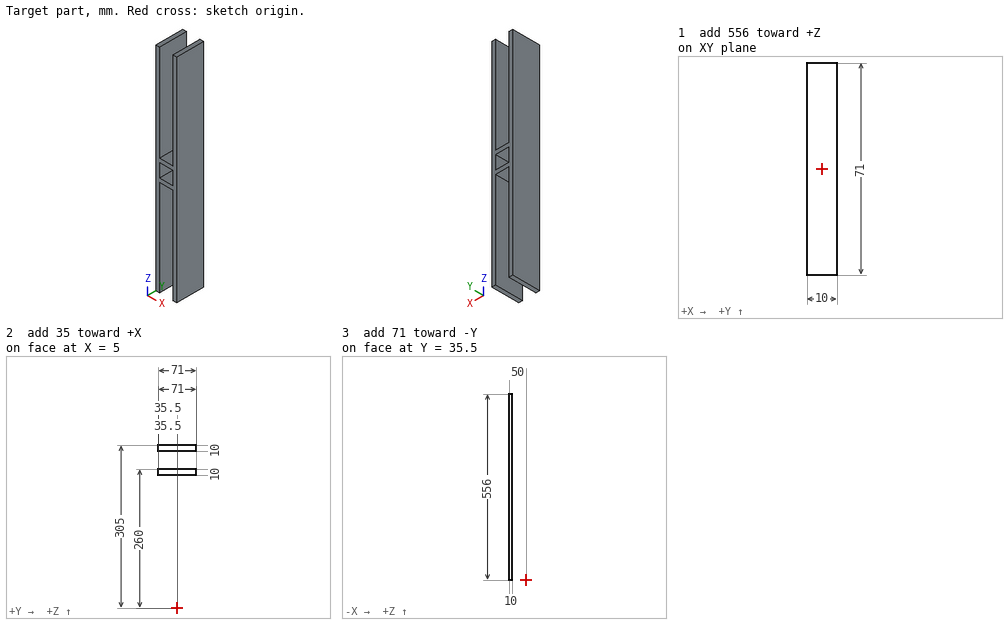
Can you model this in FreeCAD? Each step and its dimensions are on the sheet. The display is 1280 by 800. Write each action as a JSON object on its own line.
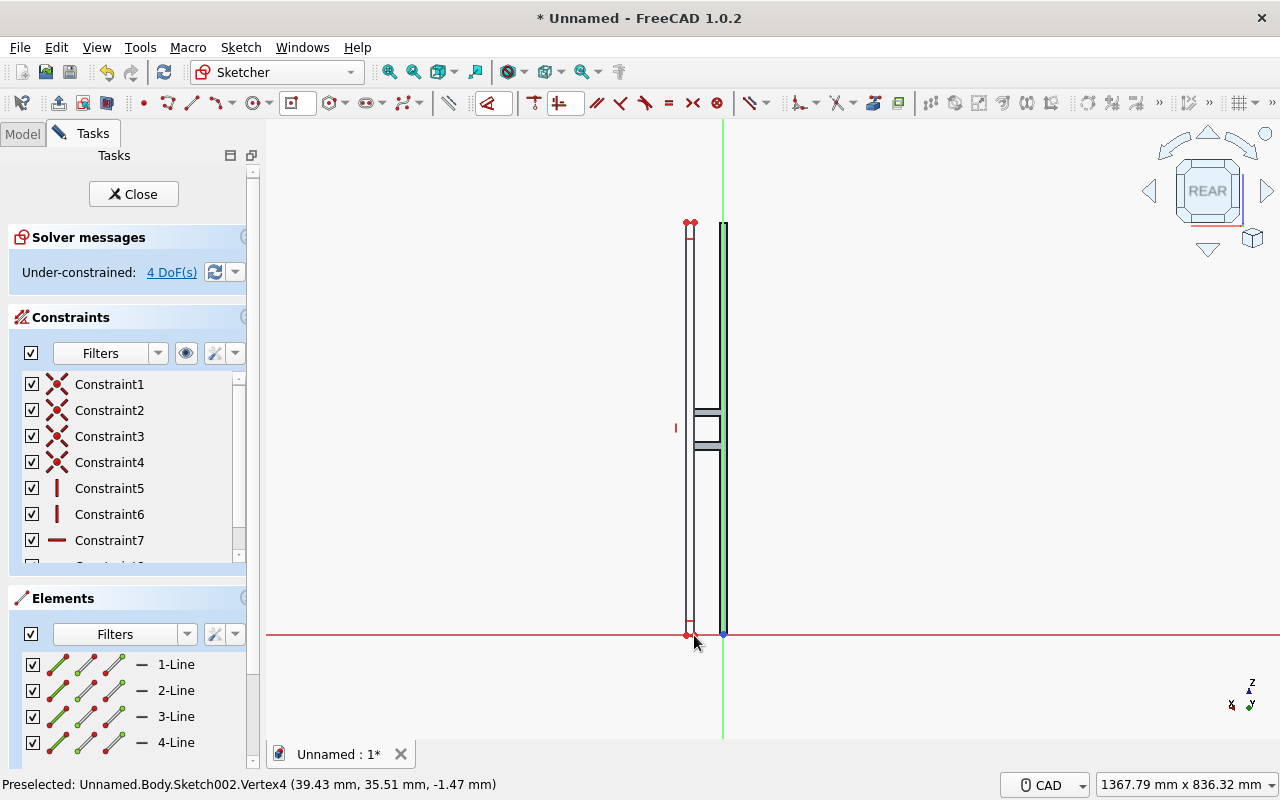
{"action": "scroll", "coordinate": [686, 636], "scroll_direction": "up", "scroll_amount": 3}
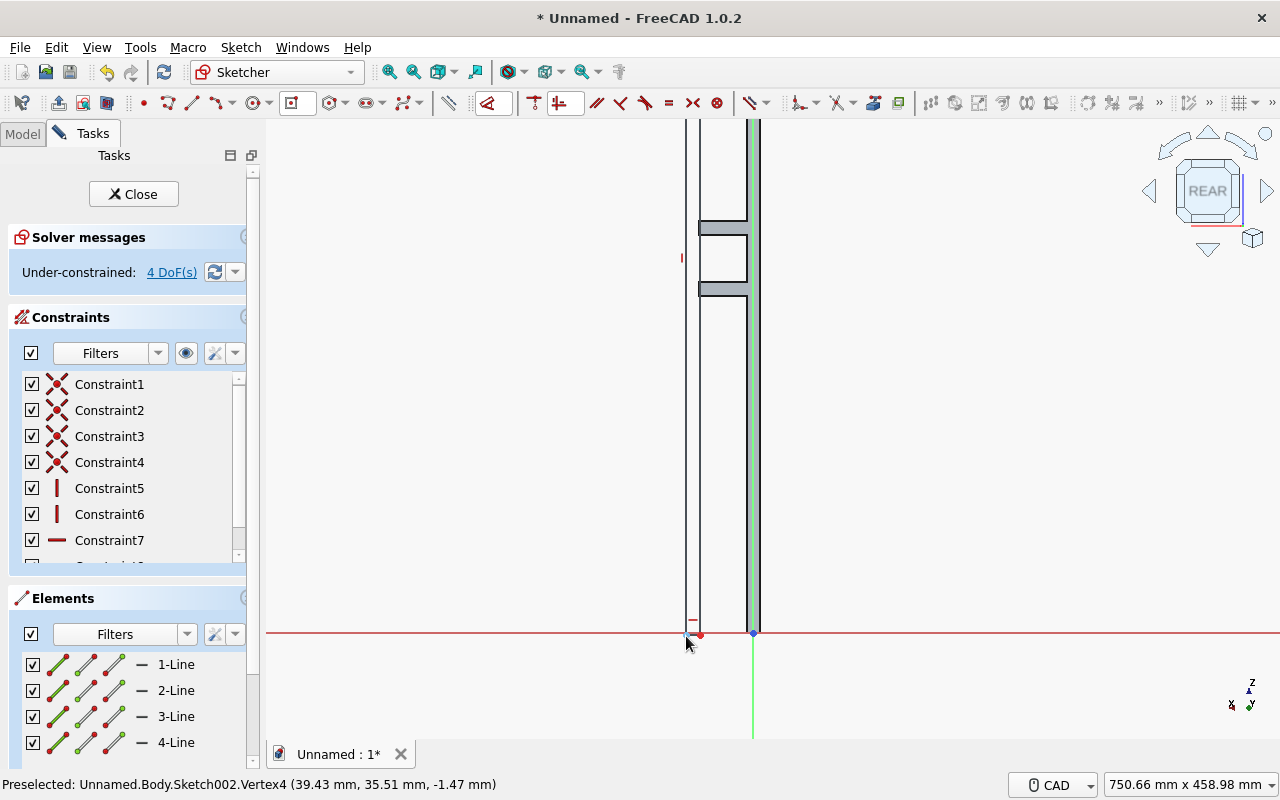
{"action": "left_click", "coordinate": [686, 635]}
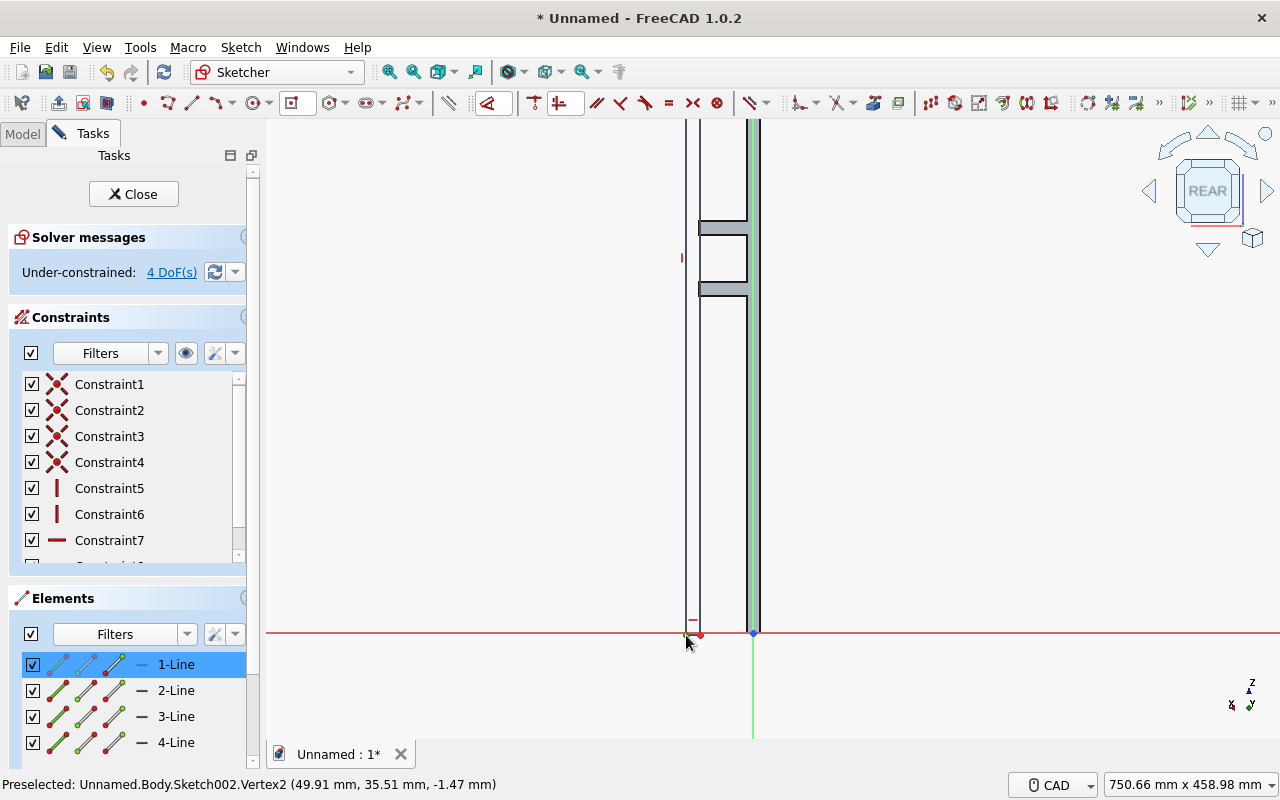
{"action": "left_click", "coordinate": [353, 633]}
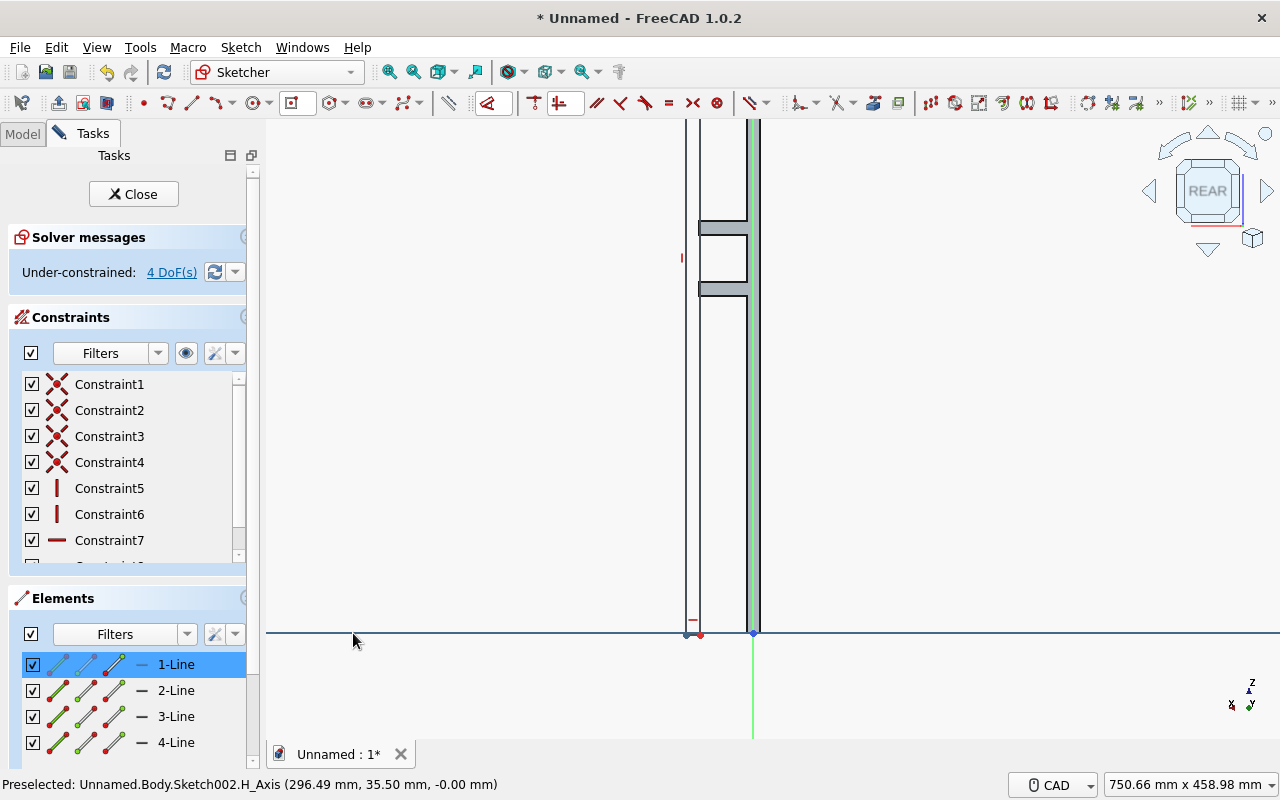
{"action": "left_click", "coordinate": [534, 104]}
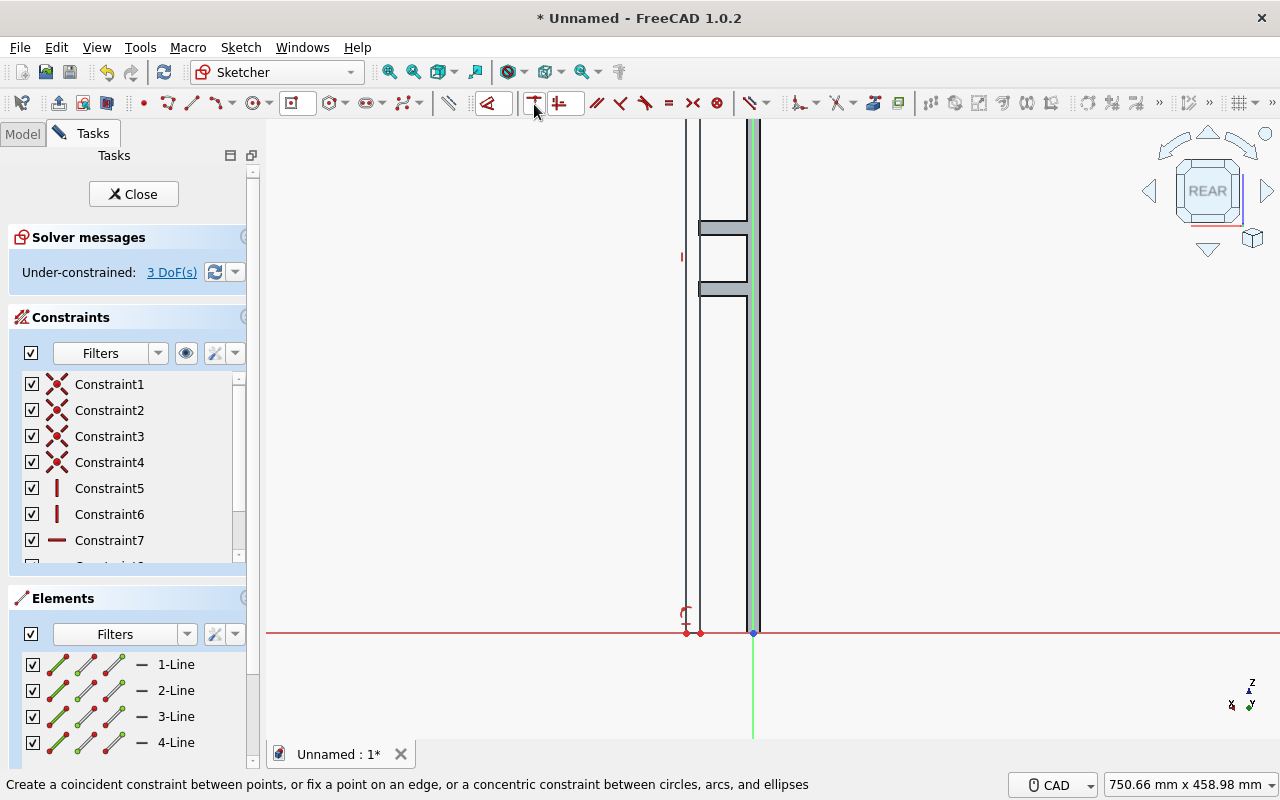
{"action": "scroll", "coordinate": [693, 633], "scroll_direction": "up", "scroll_amount": 6}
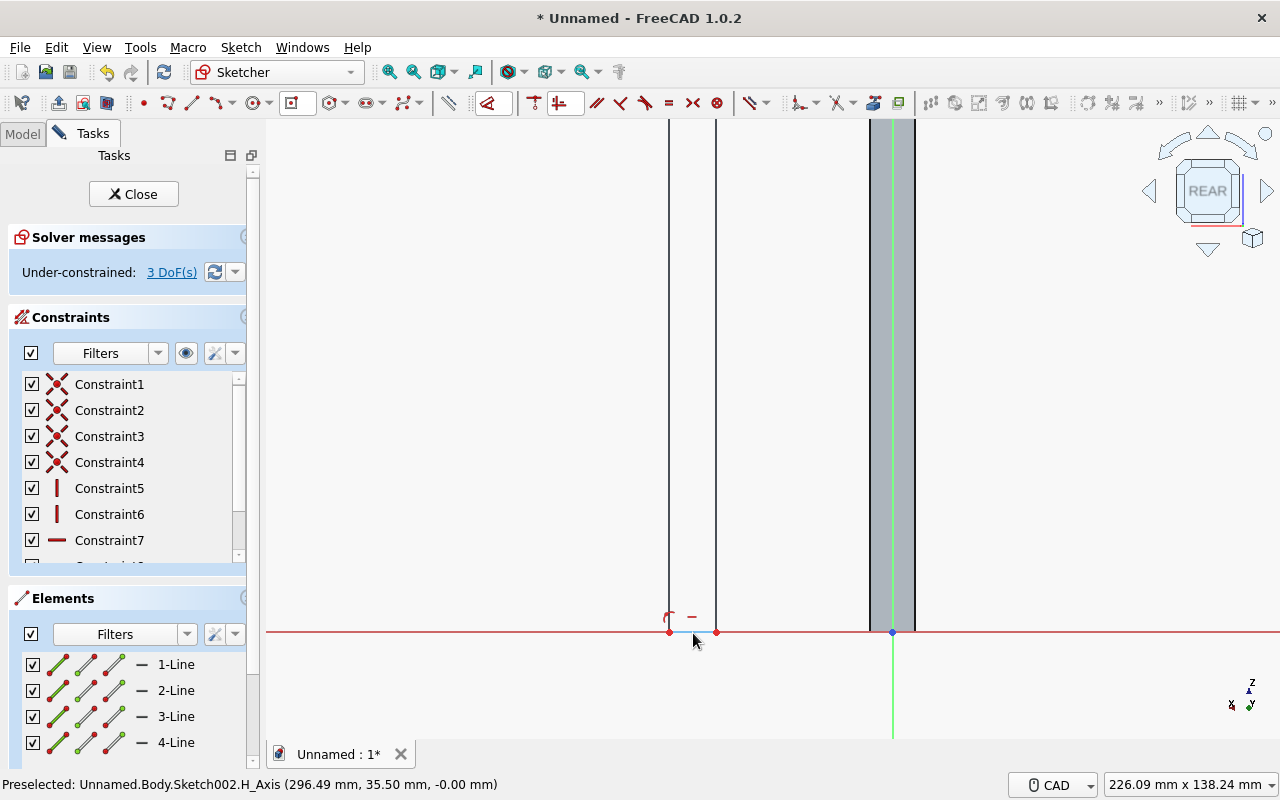
{"action": "left_click", "coordinate": [693, 632]}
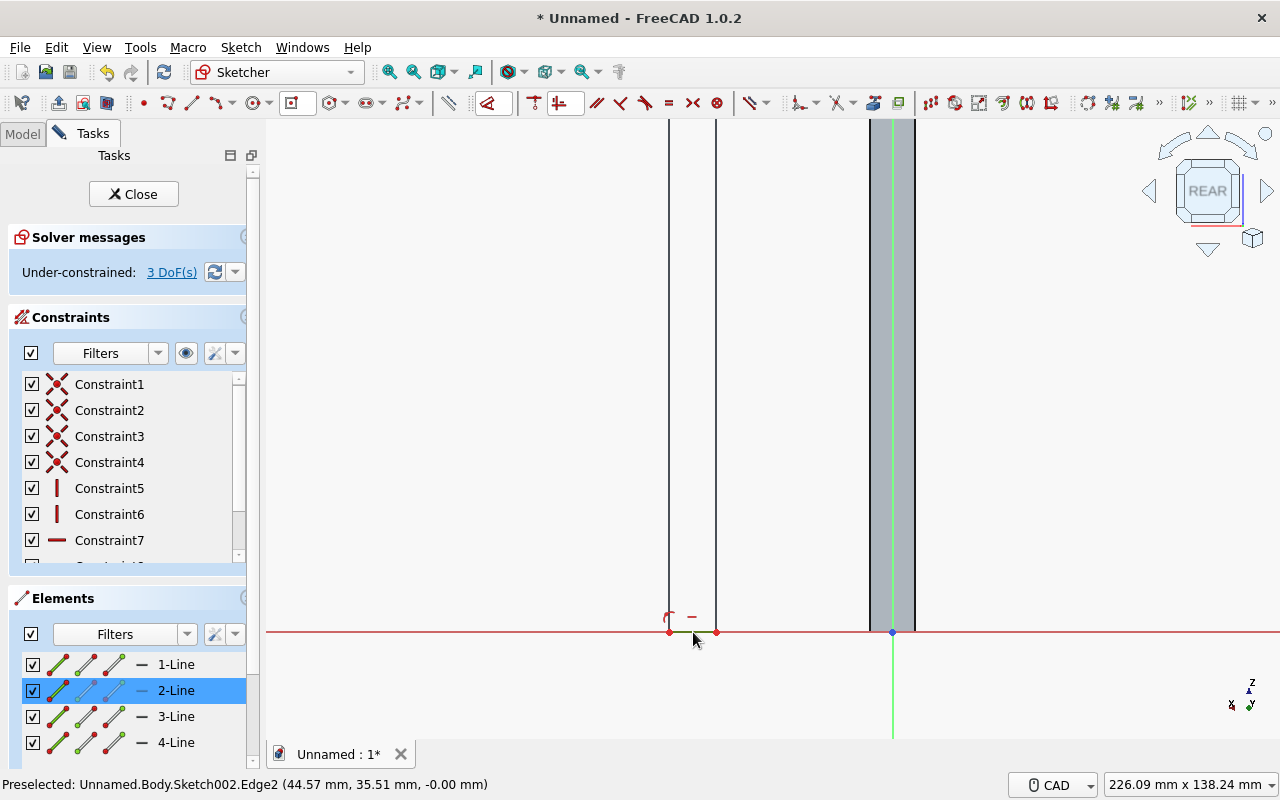
{"action": "left_click", "coordinate": [506, 104]}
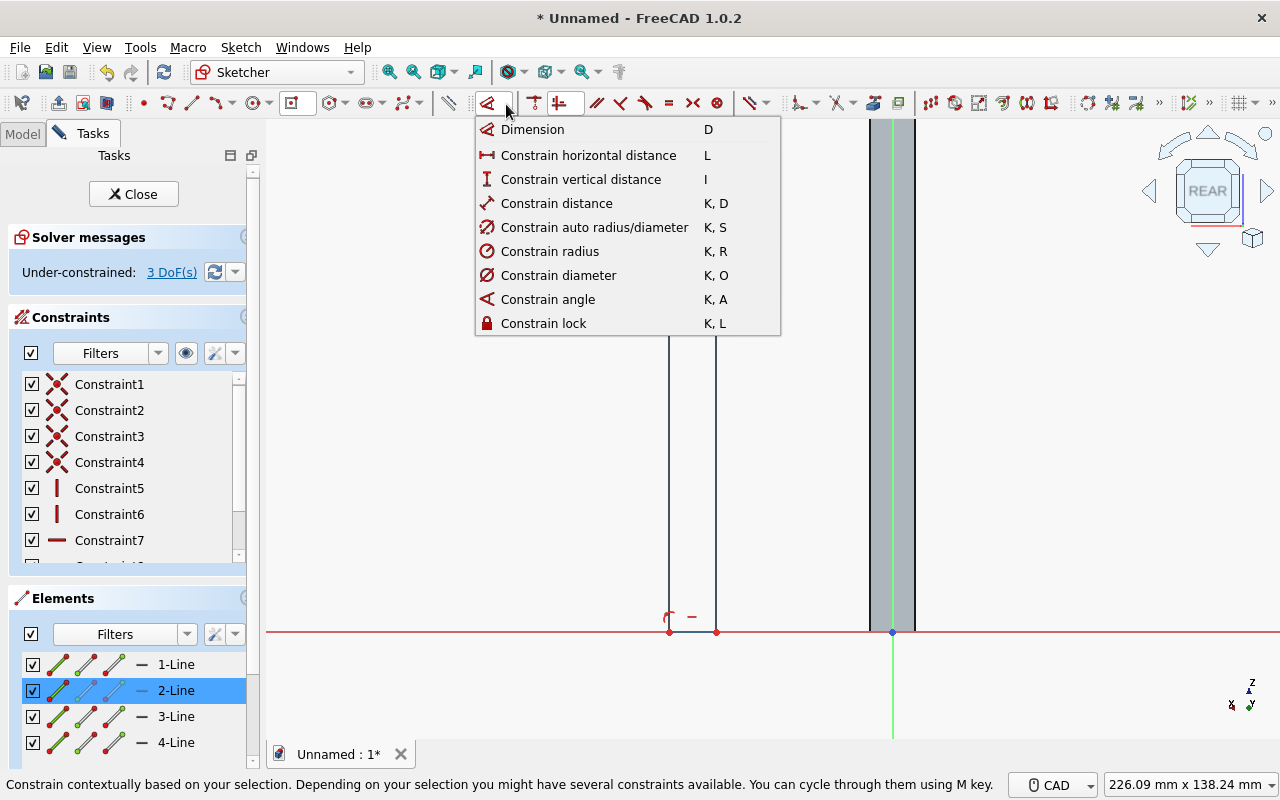
{"action": "left_click", "coordinate": [628, 155]}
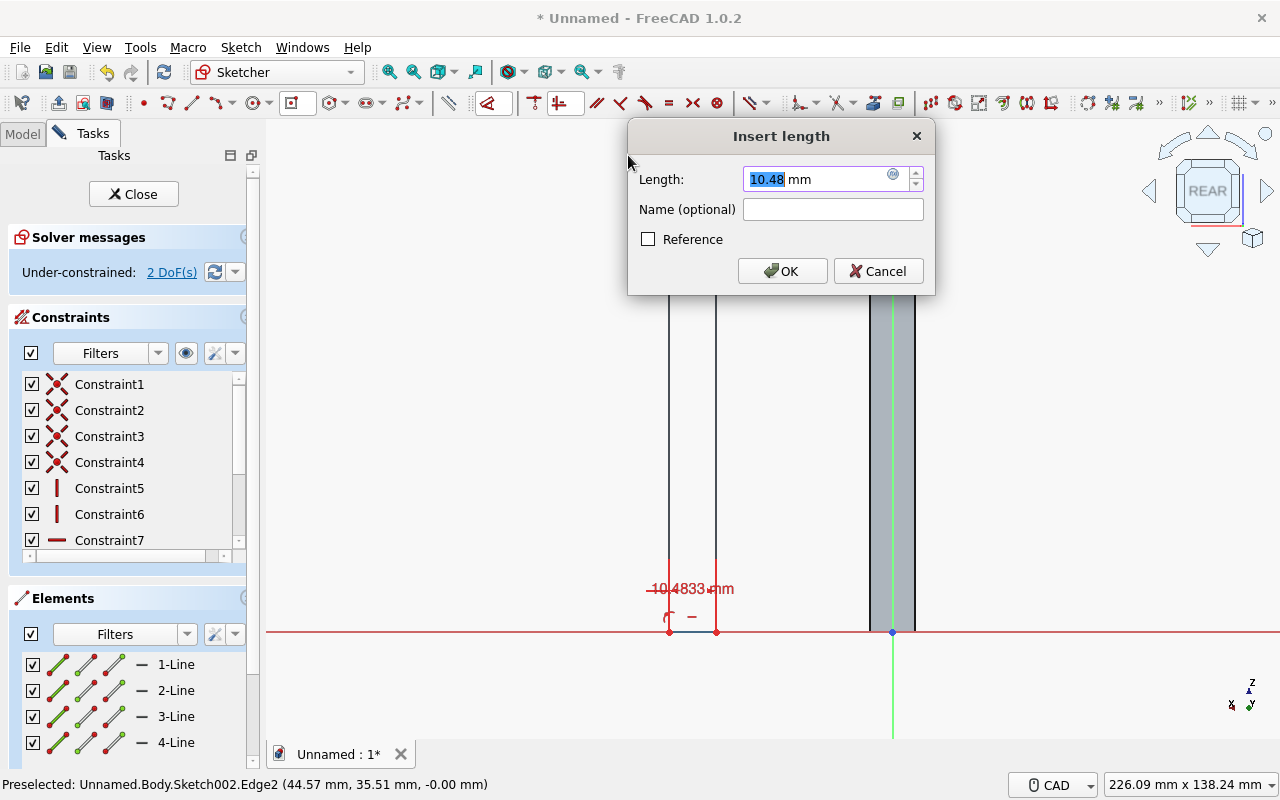
{"action": "type", "text": "10"}
{"action": "key", "text": "Return"}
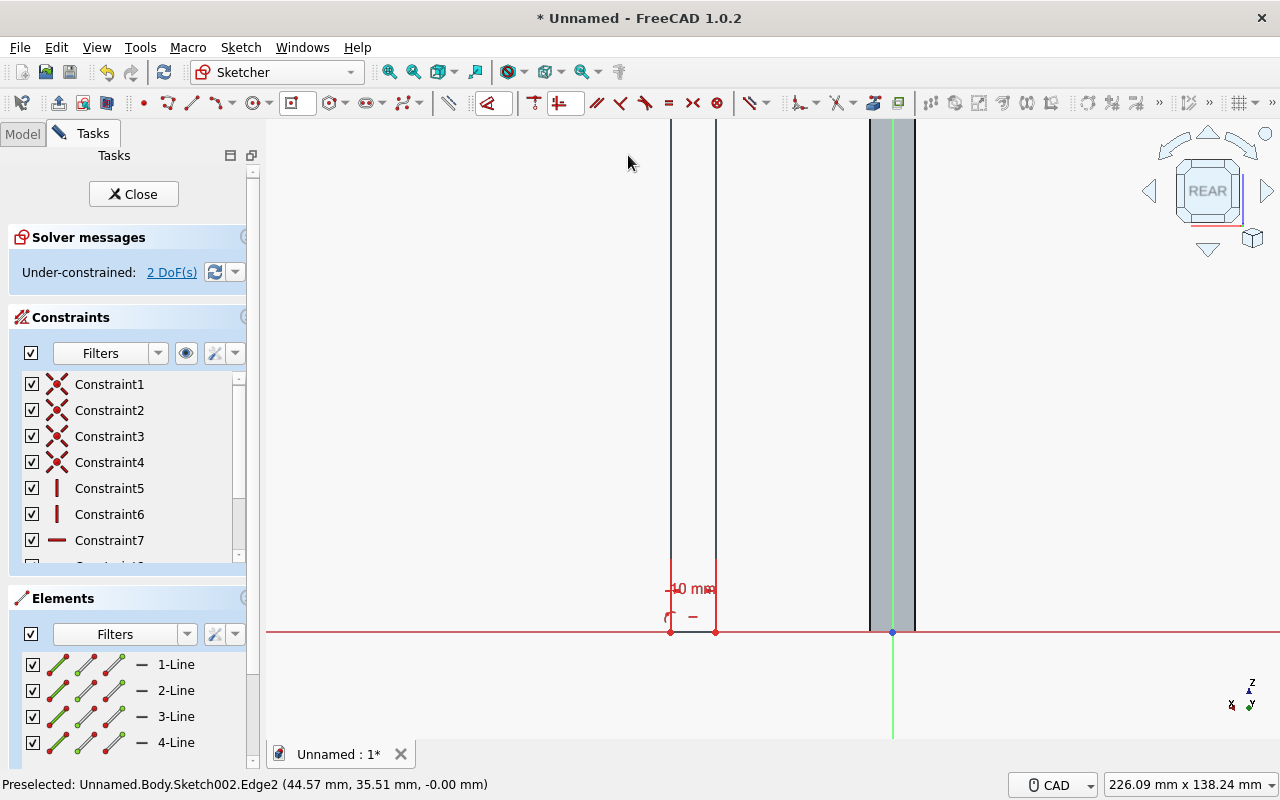
{"action": "scroll", "coordinate": [689, 636], "scroll_direction": "down", "scroll_amount": 9}